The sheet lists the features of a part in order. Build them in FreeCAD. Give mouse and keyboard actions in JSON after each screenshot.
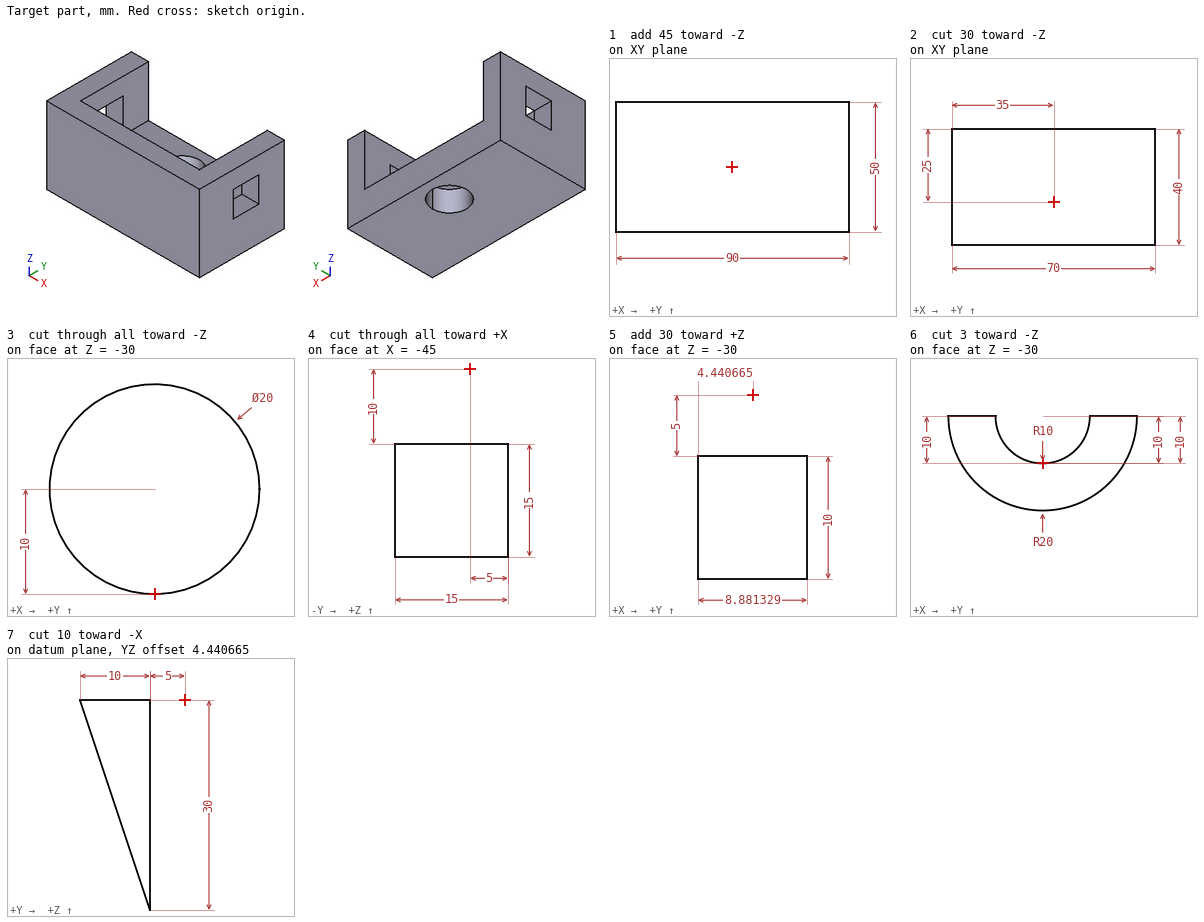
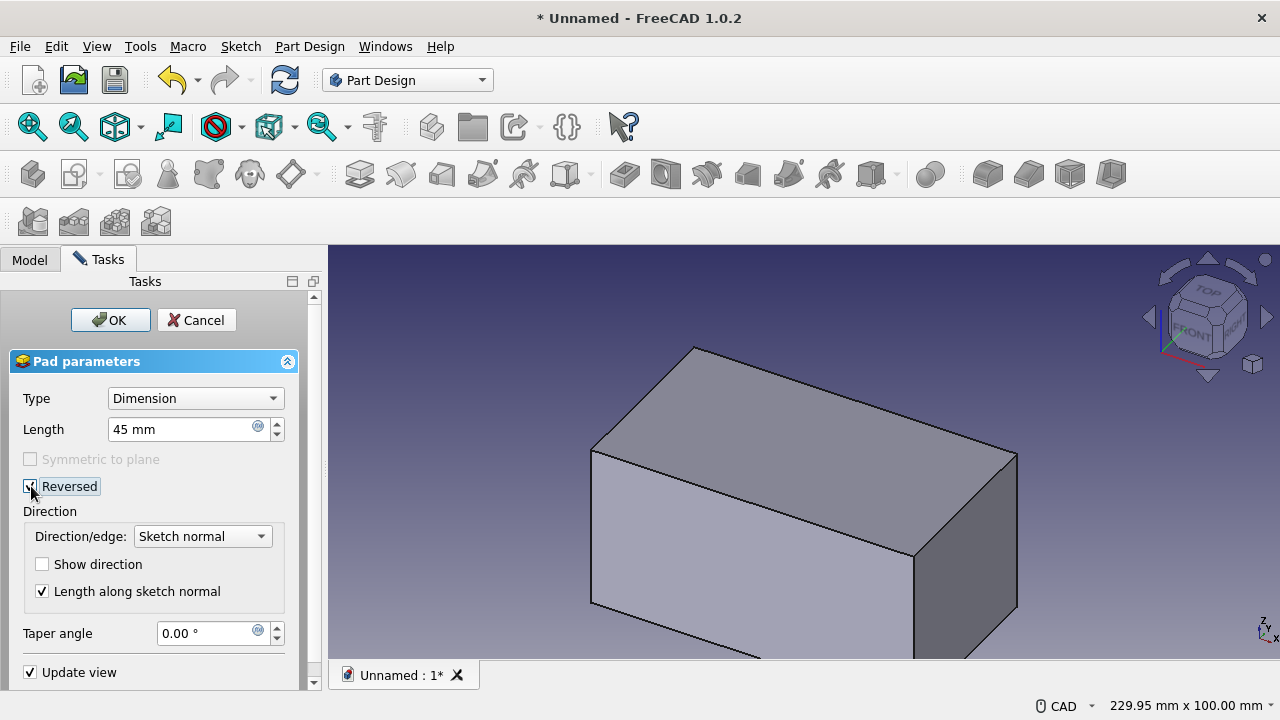
{"action": "left_click", "coordinate": [111, 320]}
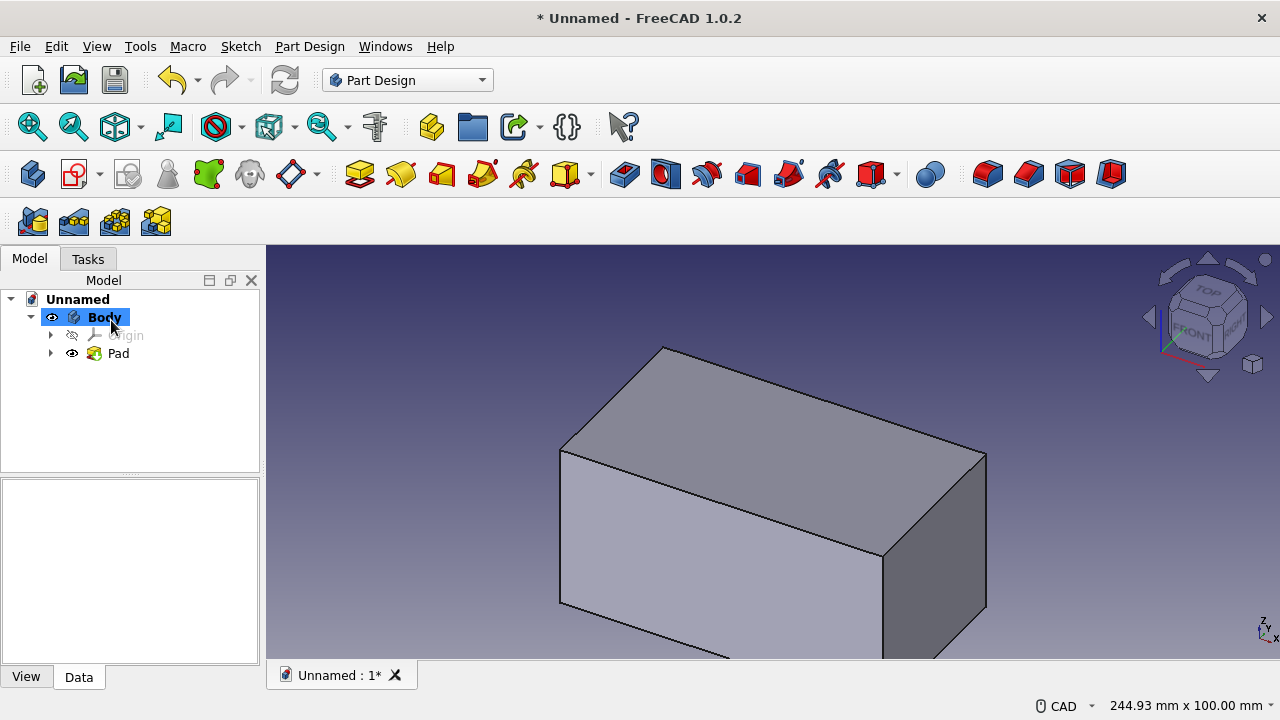
{"action": "key", "text": "v f"}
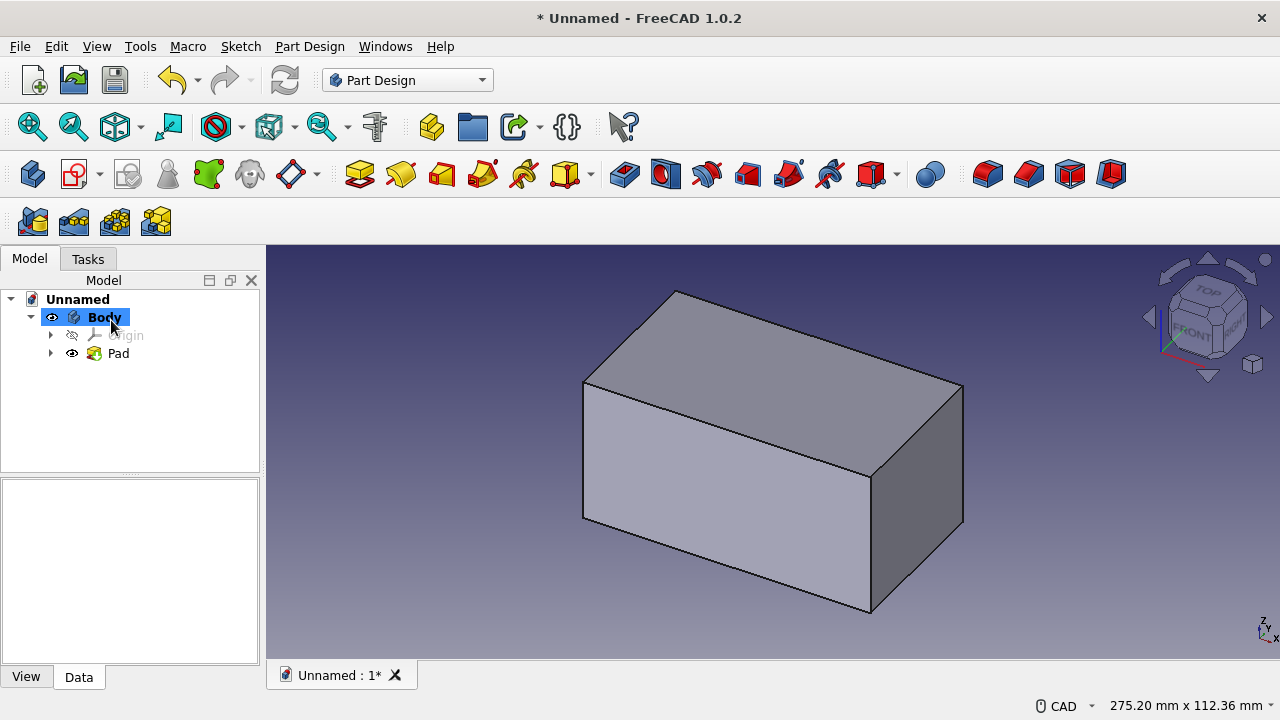
{"action": "left_click", "coordinate": [74, 174]}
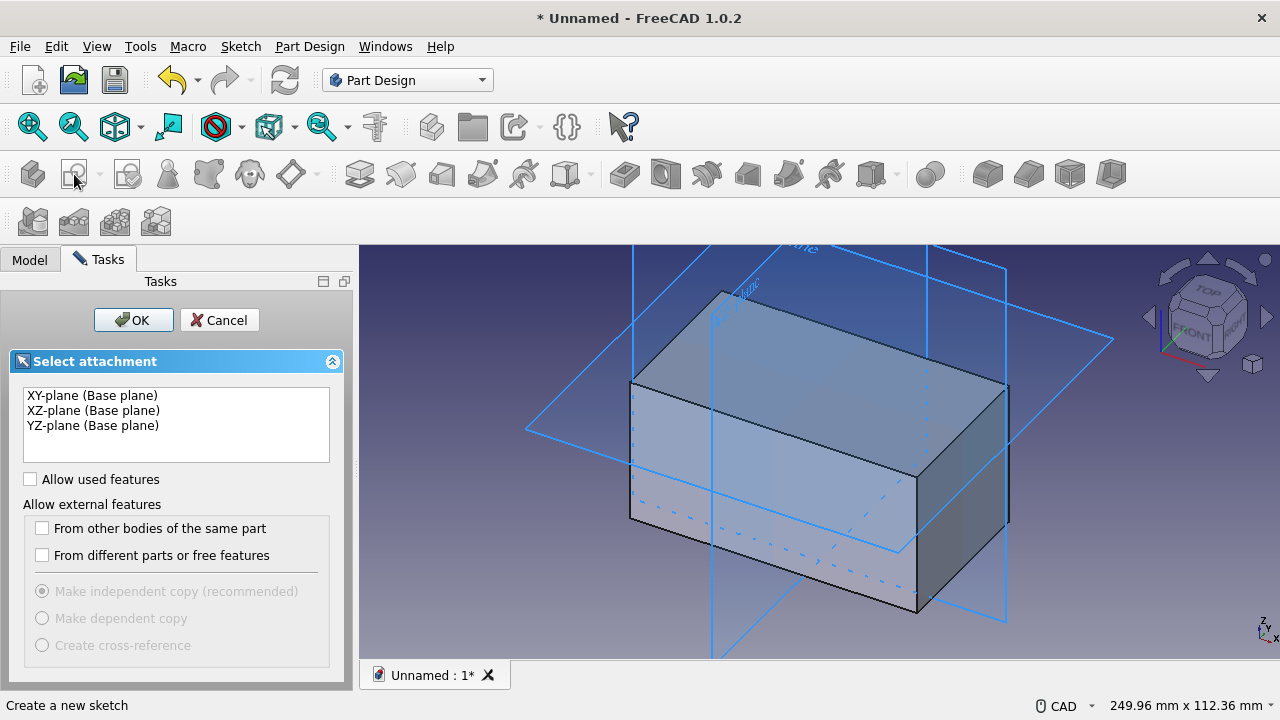
{"action": "left_click", "coordinate": [84, 396]}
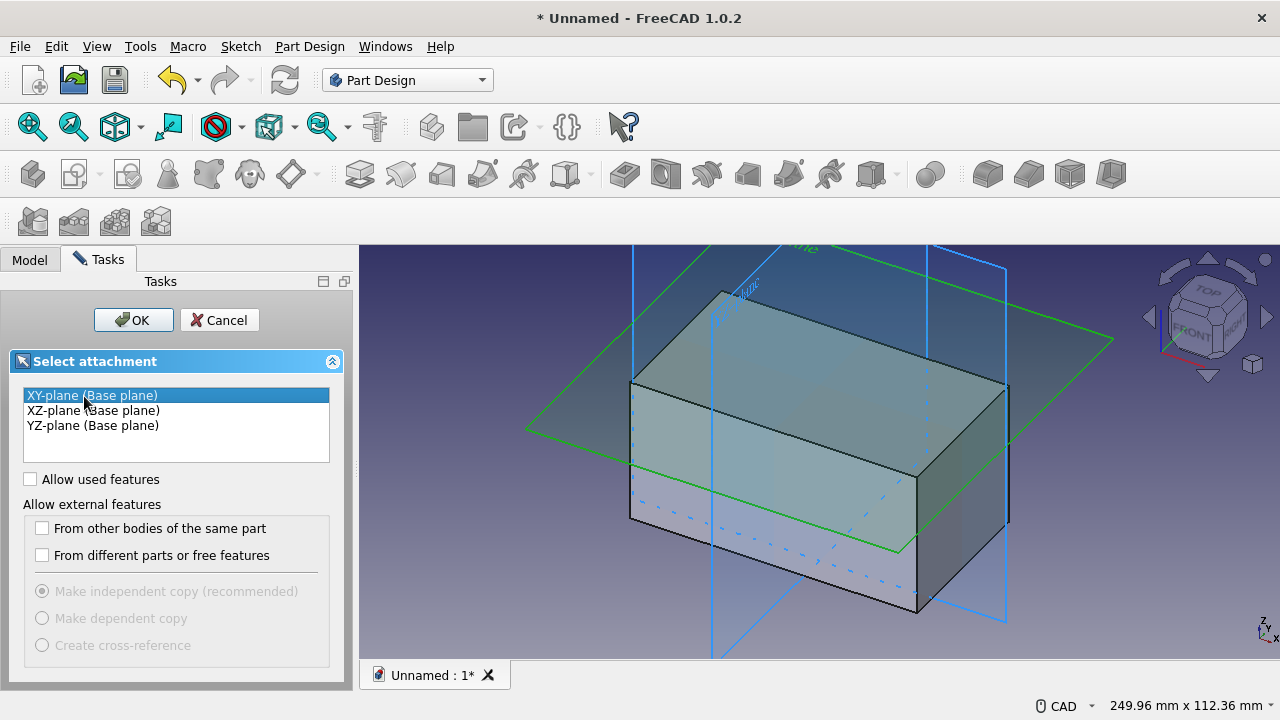
{"action": "left_click", "coordinate": [134, 320]}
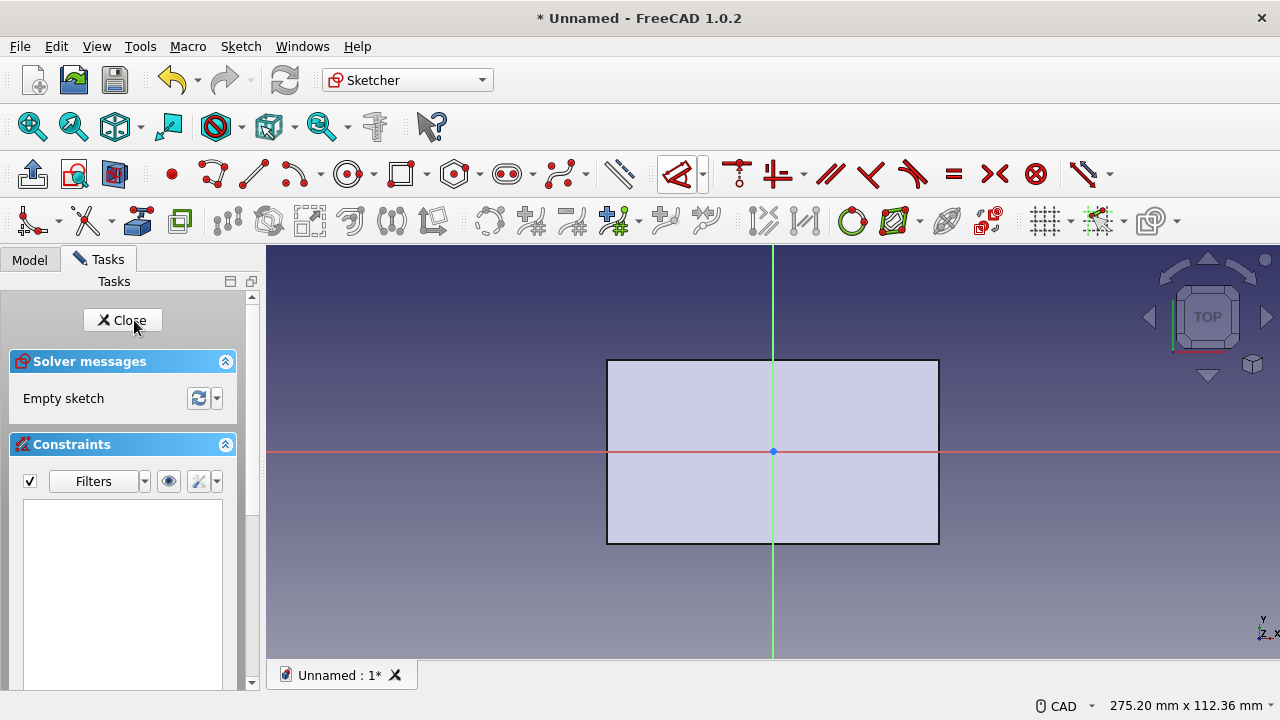
{"action": "scroll", "coordinate": [856, 411], "scroll_direction": "up", "scroll_amount": 3}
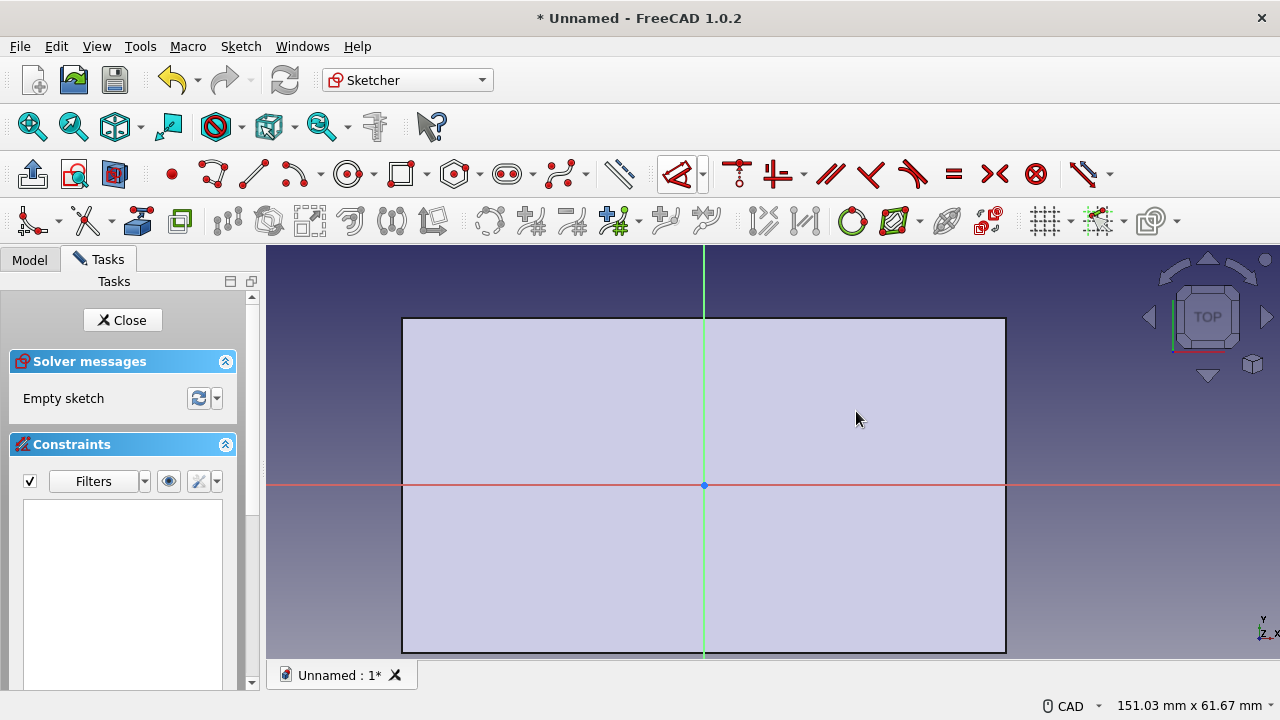
{"action": "key", "text": "g r"}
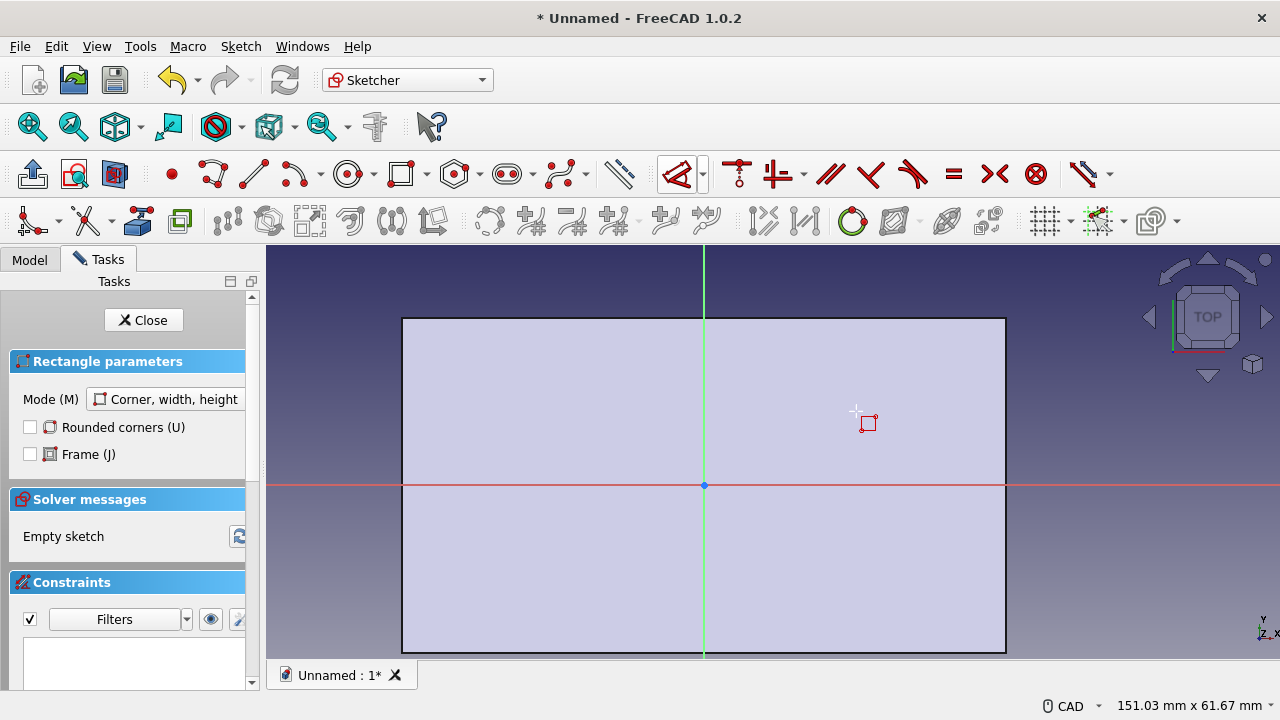
{"action": "left_click", "coordinate": [469, 318]}
{"action": "mouse_move", "coordinate": [939, 586]}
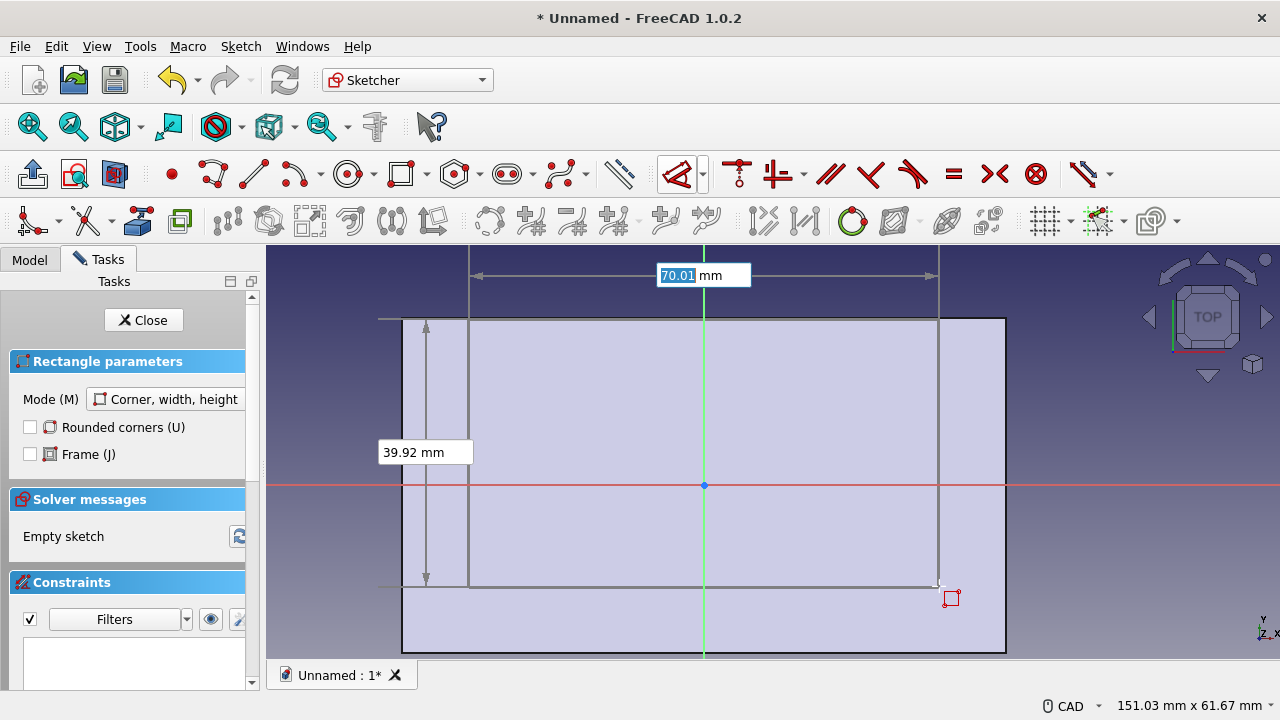
{"action": "type", "text": "70"}
{"action": "key", "text": "Tab"}
{"action": "type", "text": "40"}
{"action": "key", "text": "Return"}
{"action": "key", "text": "Escape"}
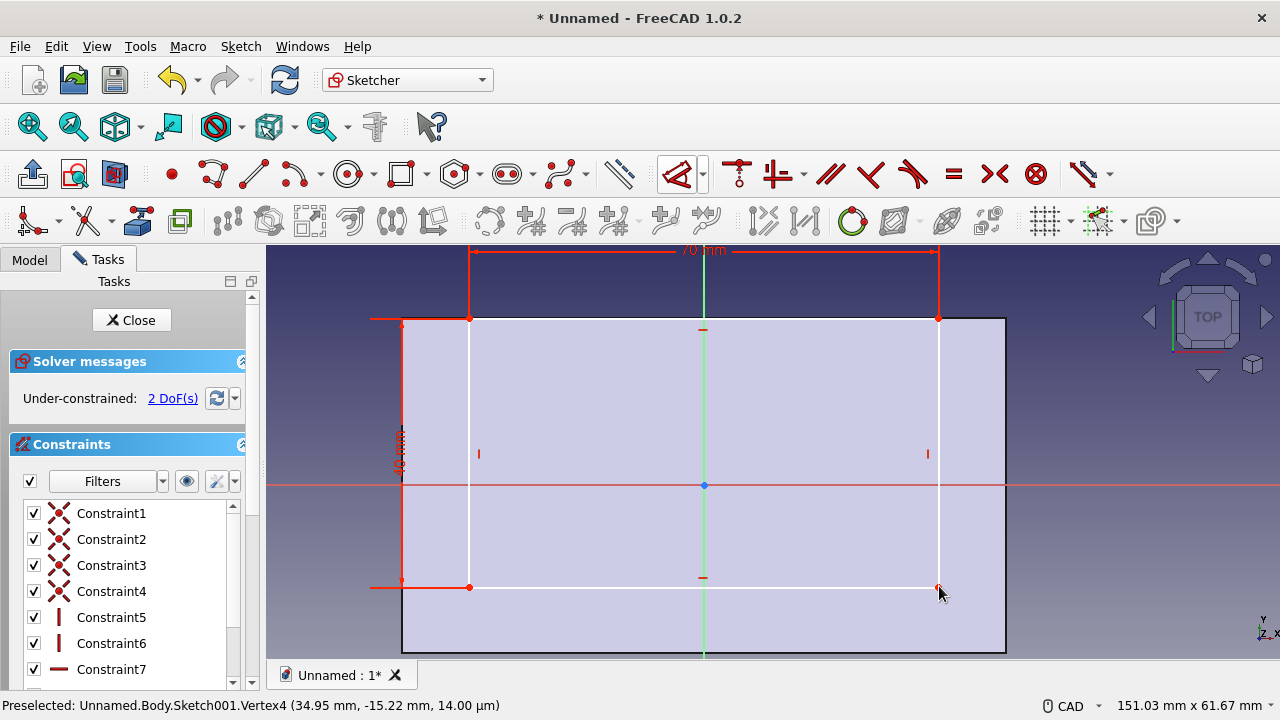
{"action": "left_click", "coordinate": [469, 319]}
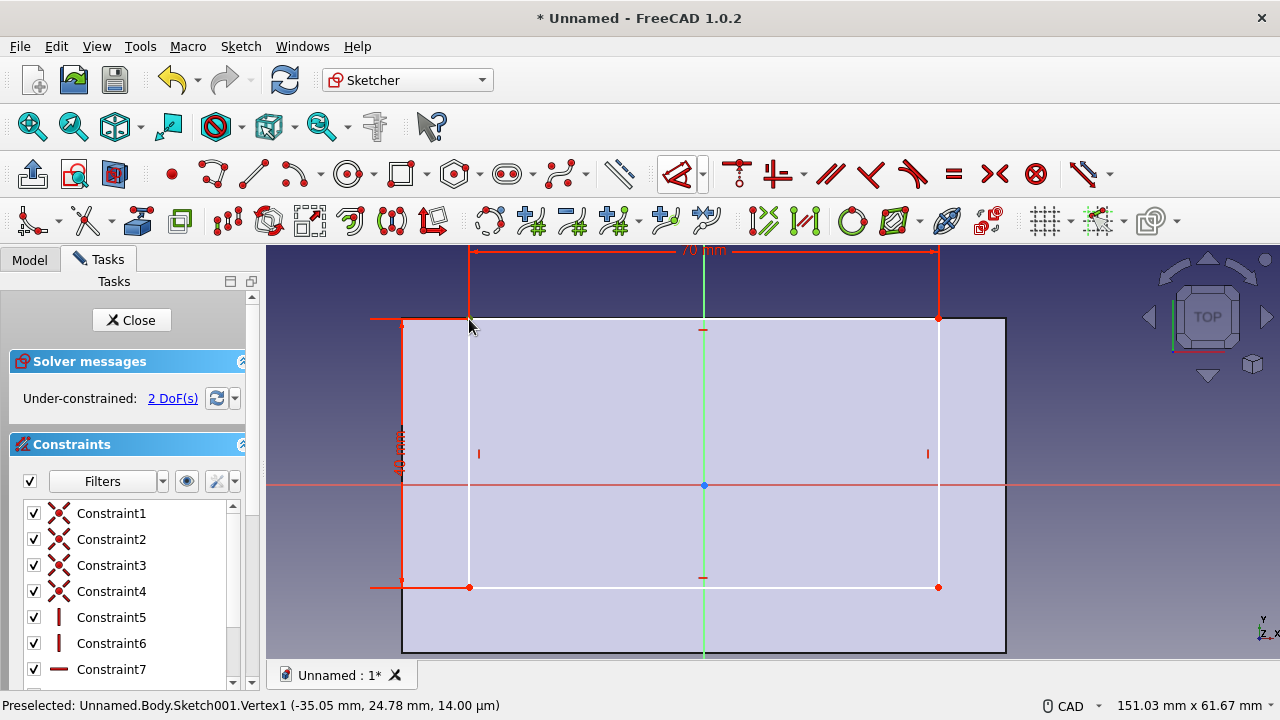
{"action": "left_click", "coordinate": [702, 174]}